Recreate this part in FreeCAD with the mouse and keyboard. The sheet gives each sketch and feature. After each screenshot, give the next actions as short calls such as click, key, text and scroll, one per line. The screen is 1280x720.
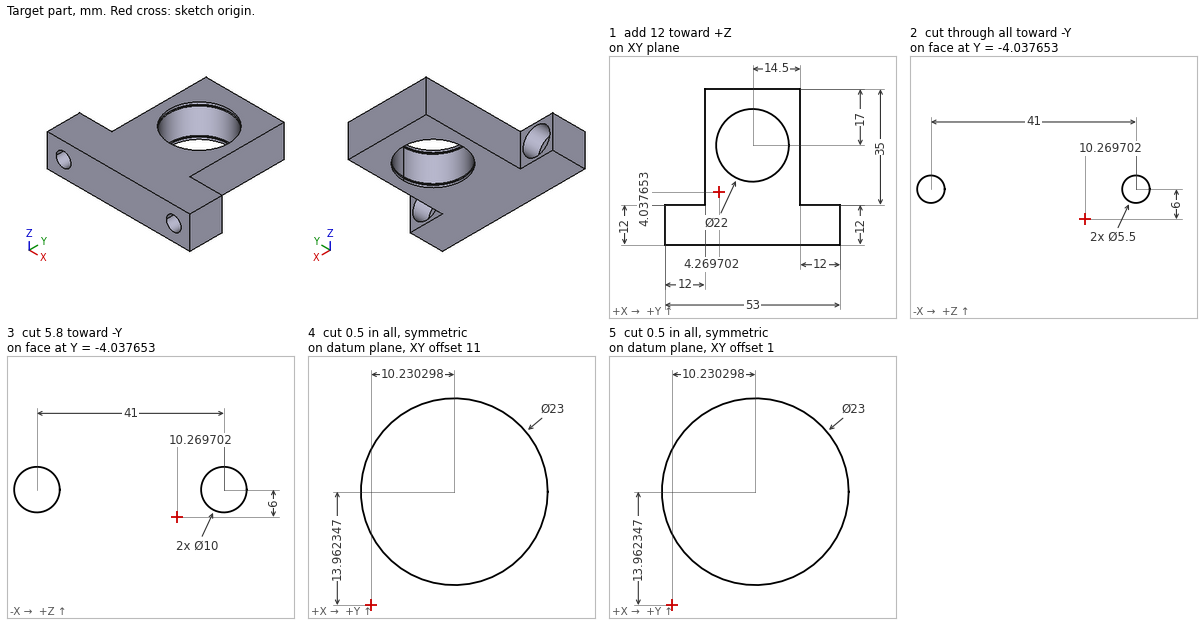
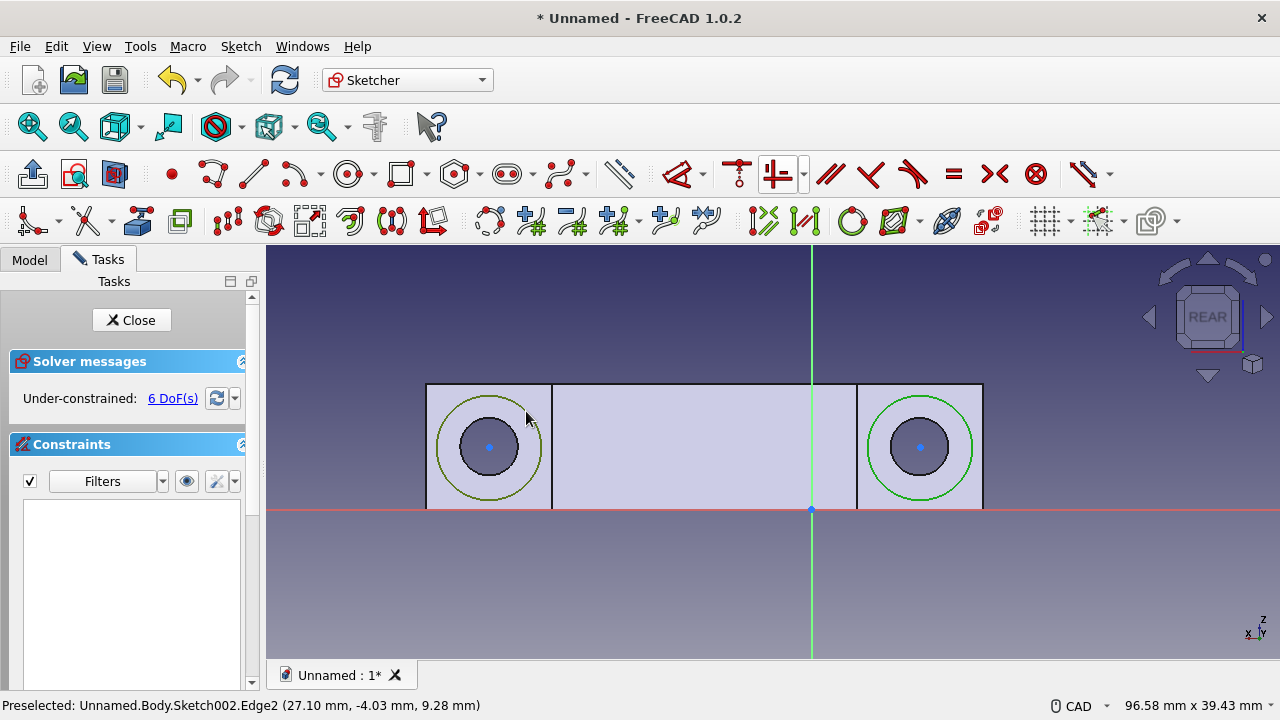
click(954, 174)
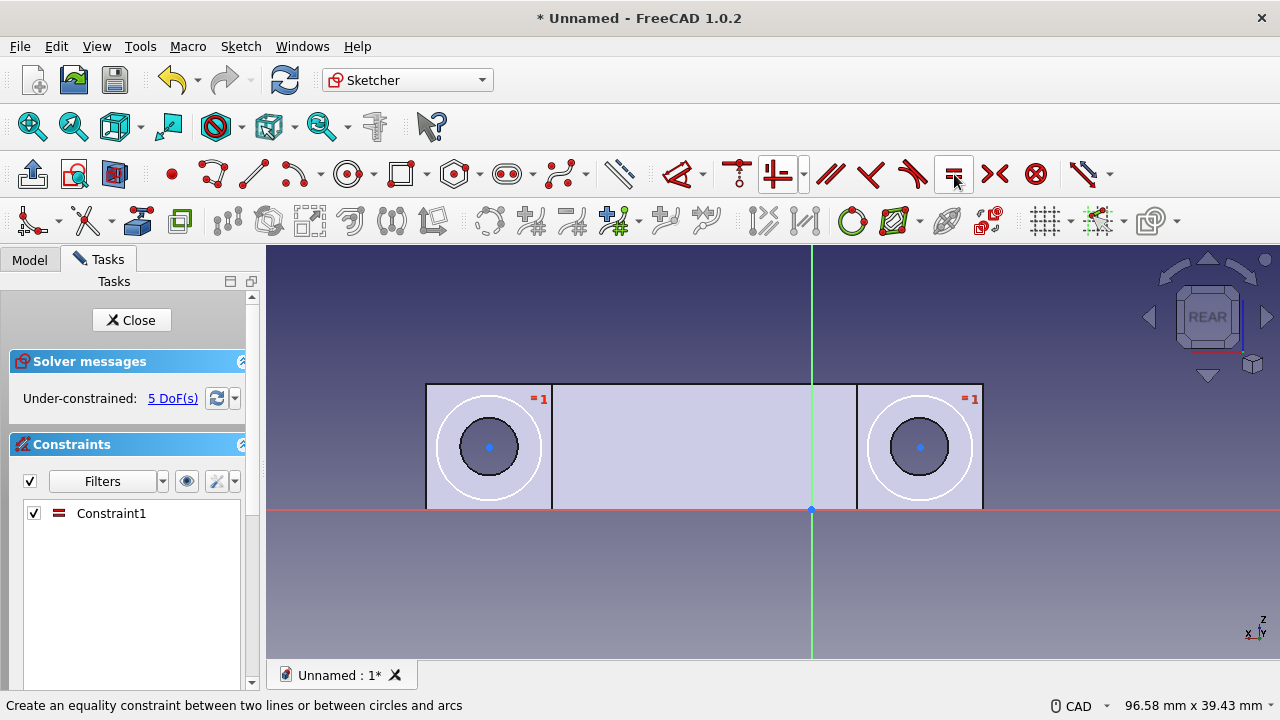
click(920, 448)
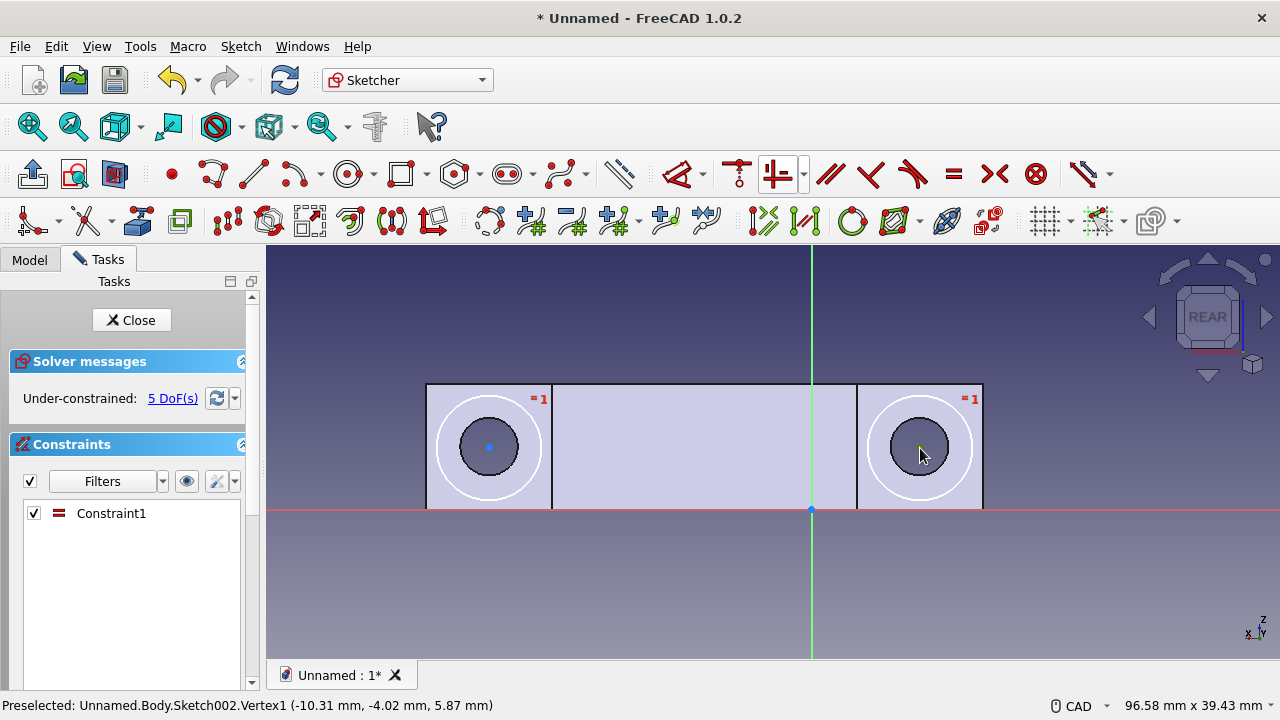
click(489, 448)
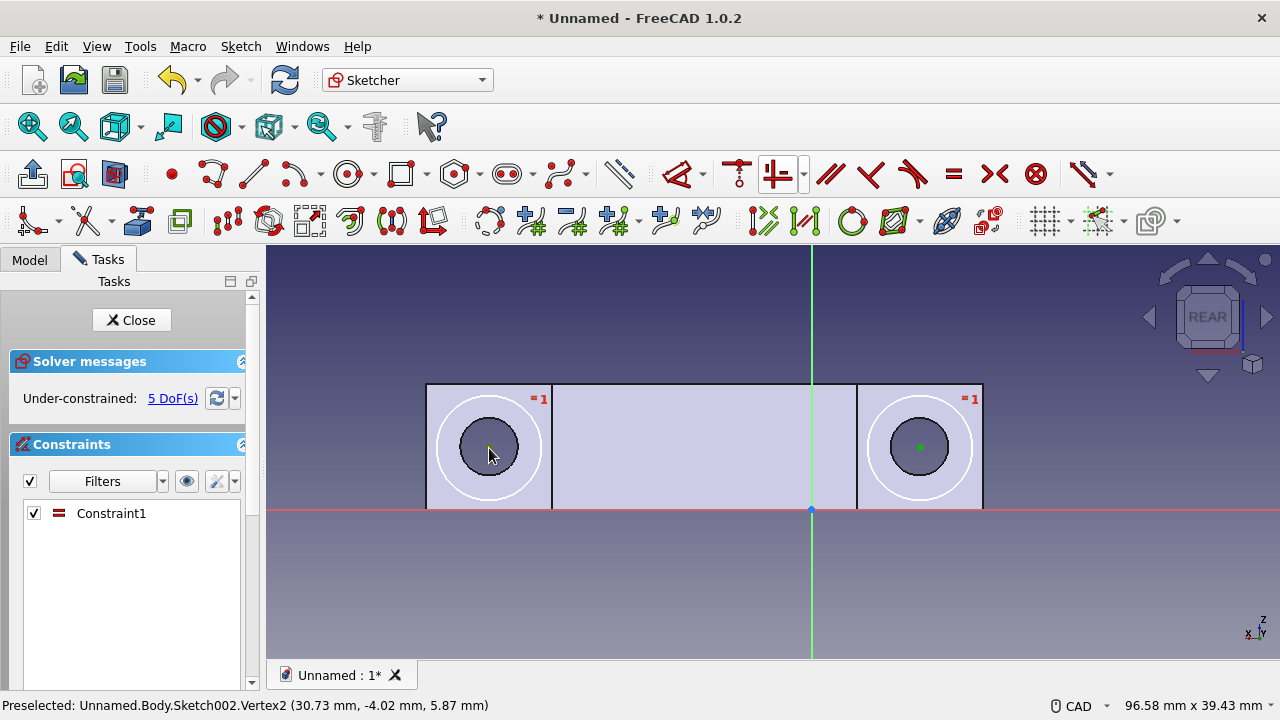
click(804, 174)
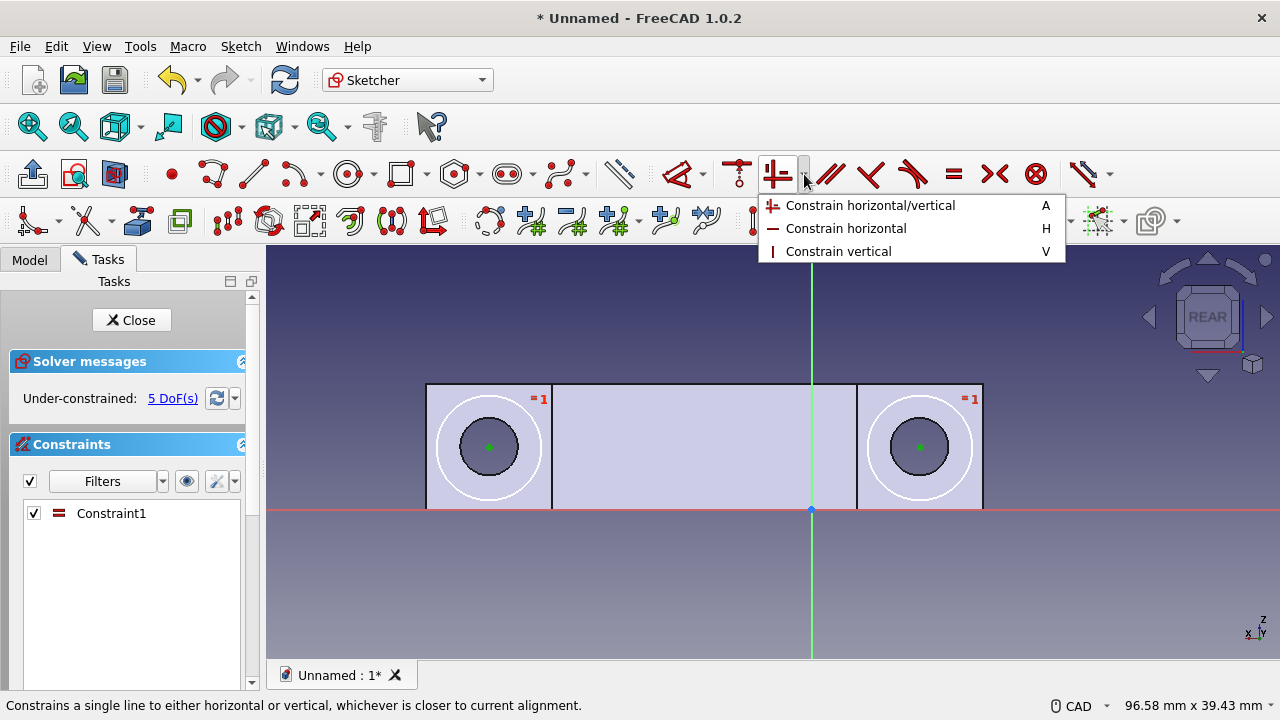
click(912, 228)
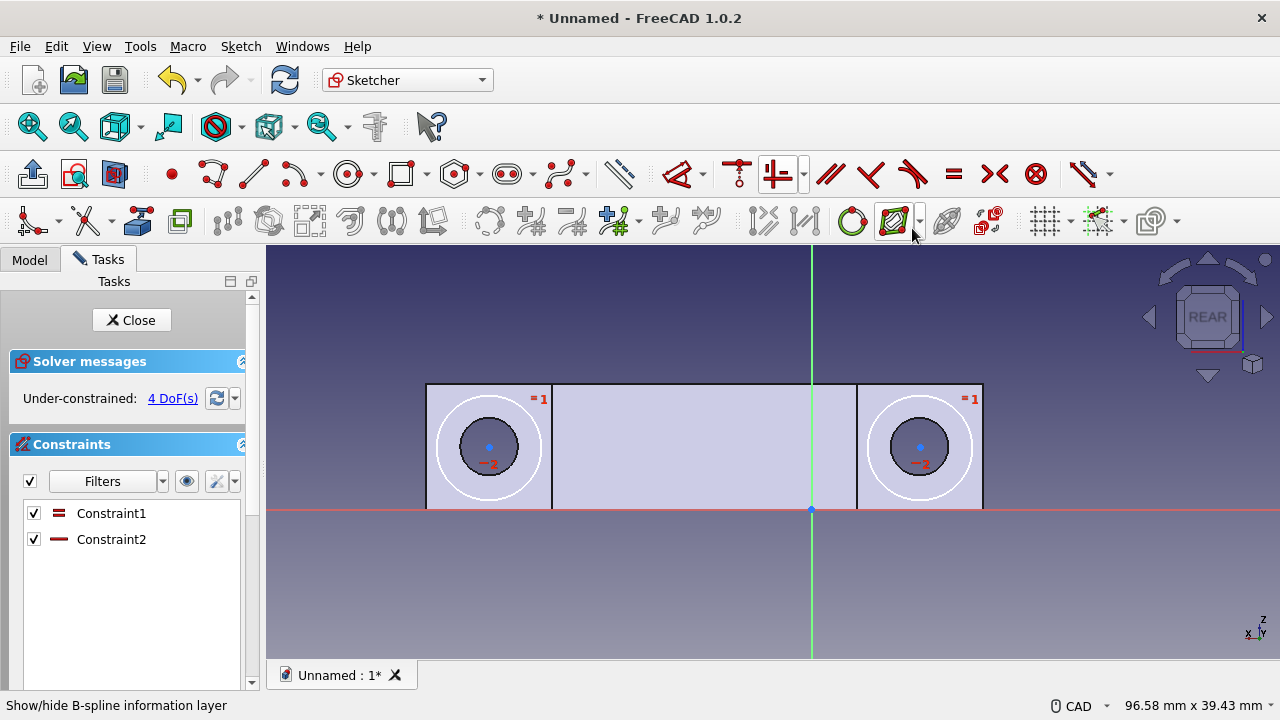
click(676, 174)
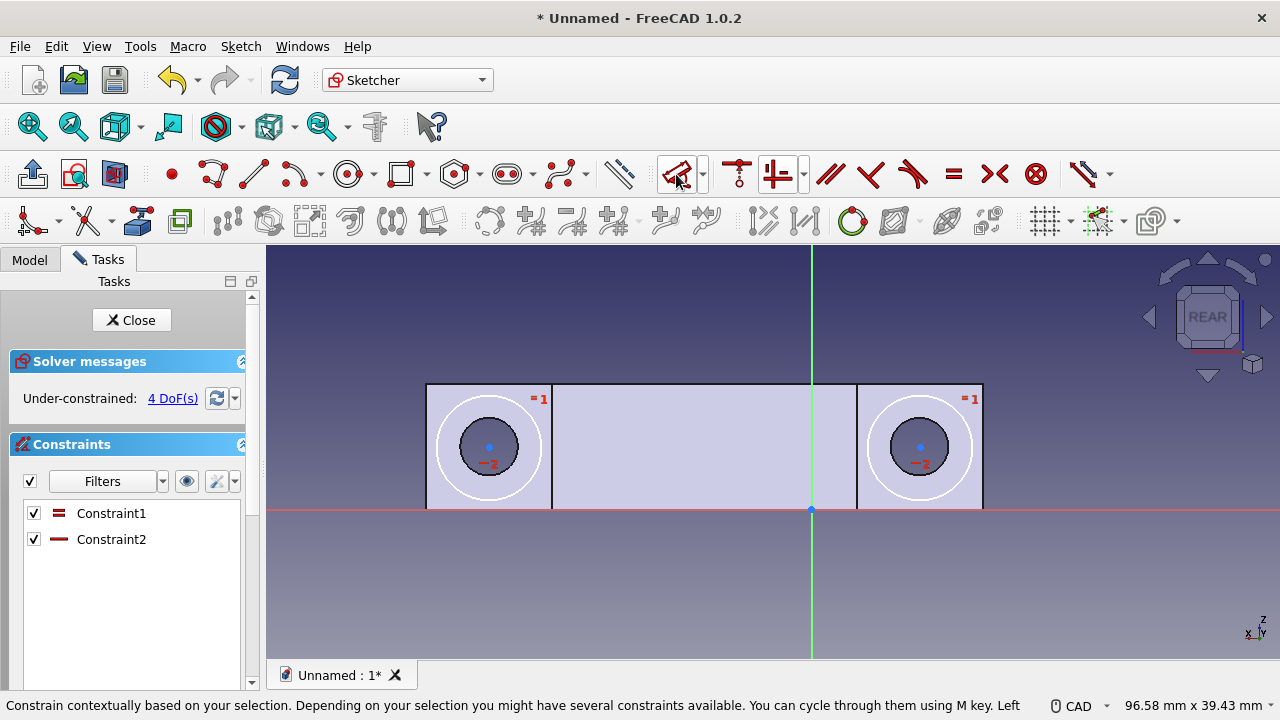
click(957, 411)
click(980, 388)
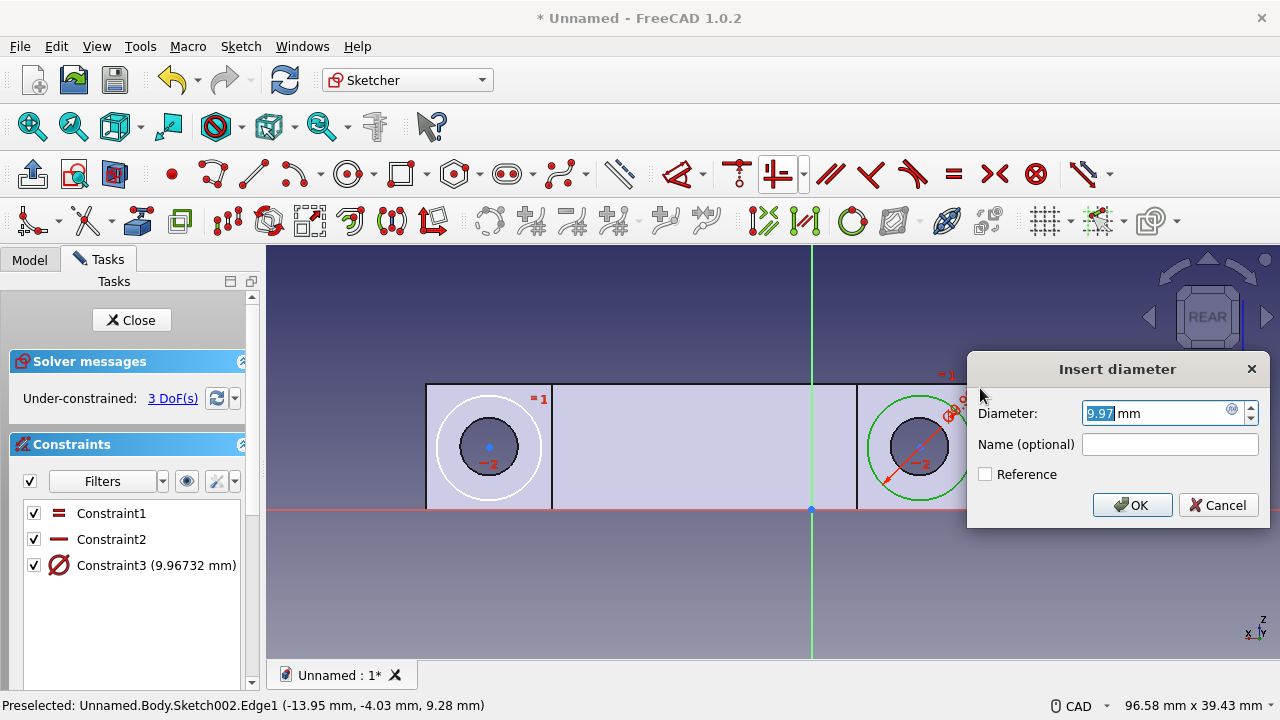
text(10)
key(Return)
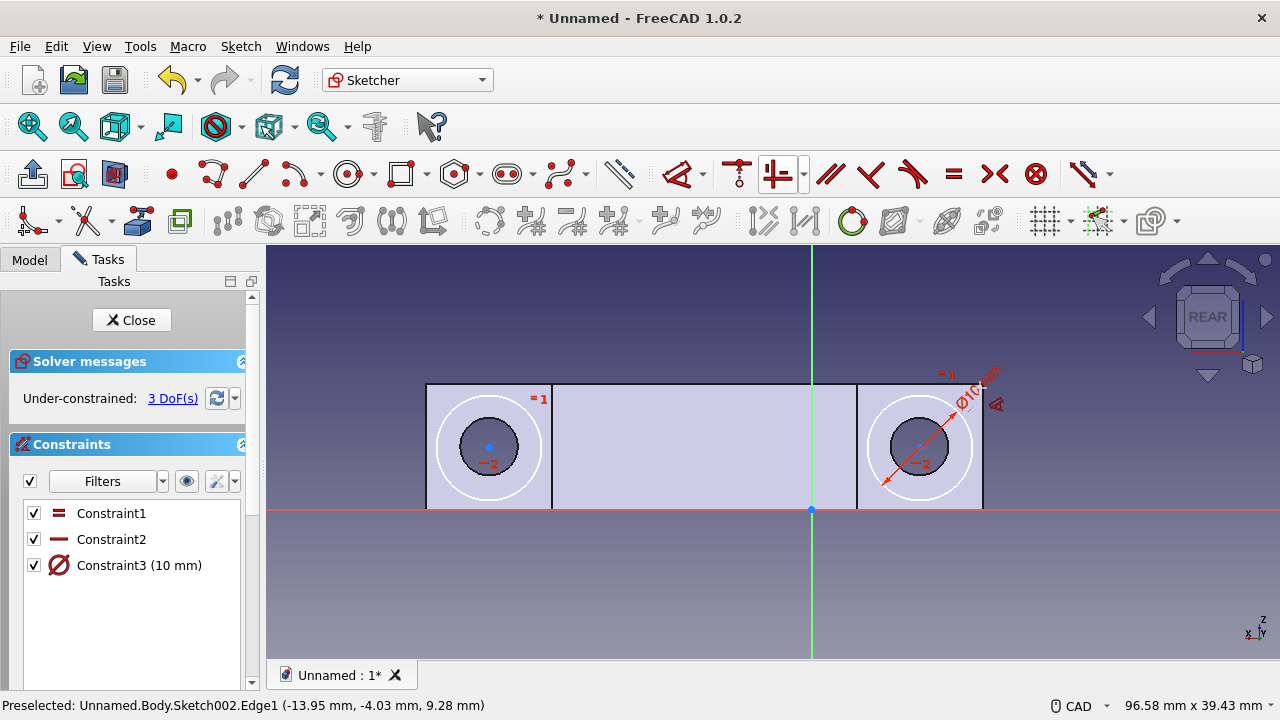
click(920, 448)
click(954, 465)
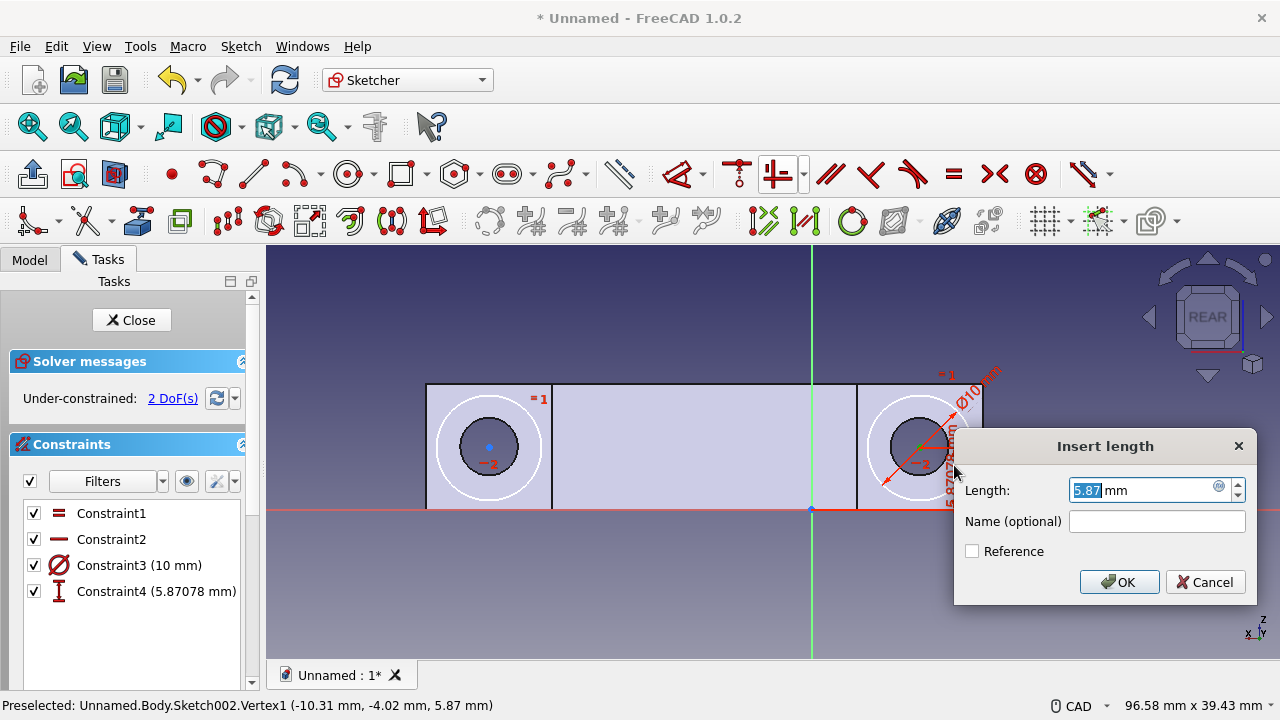
text(6)
key(Return)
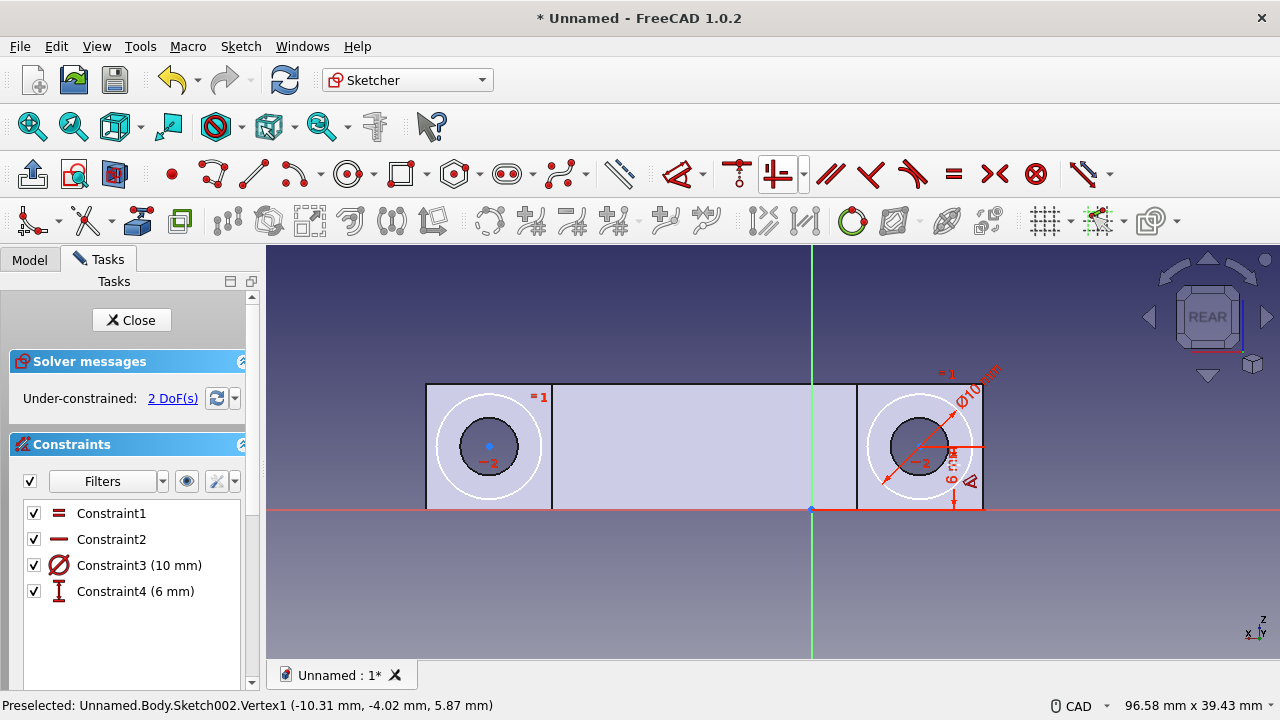
click(920, 447)